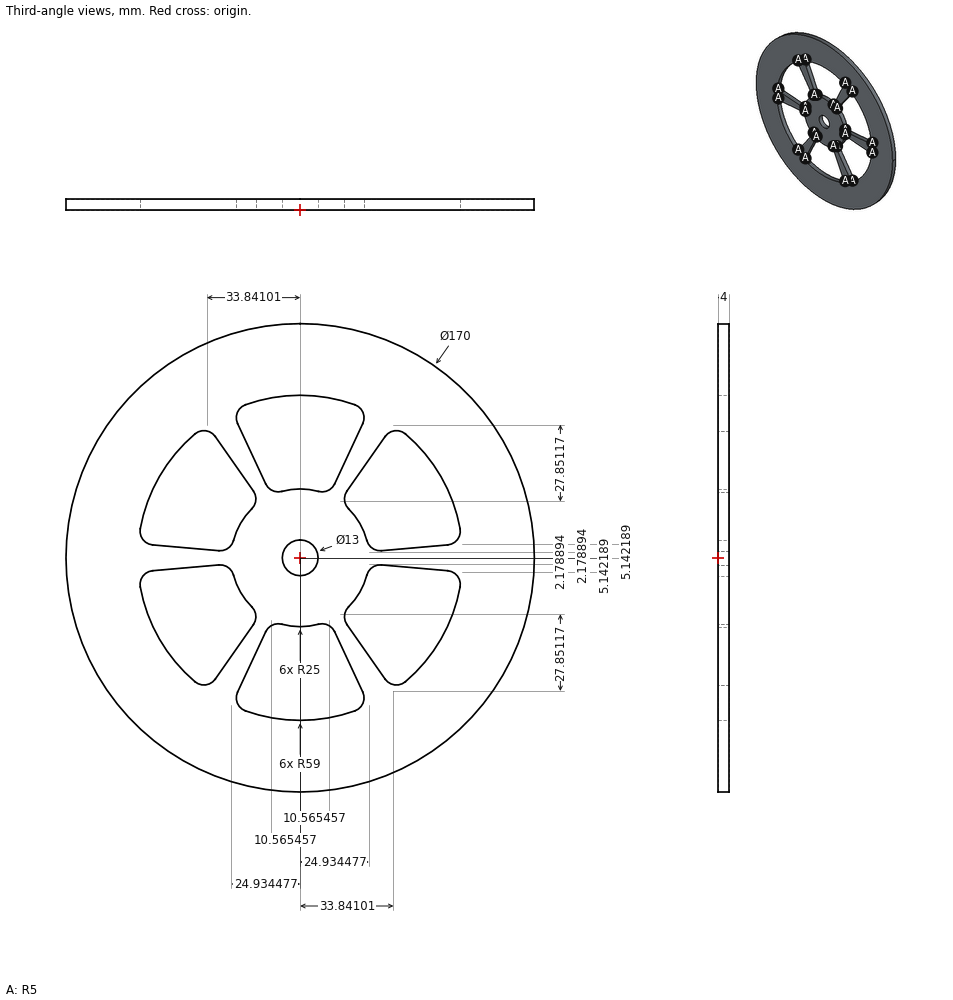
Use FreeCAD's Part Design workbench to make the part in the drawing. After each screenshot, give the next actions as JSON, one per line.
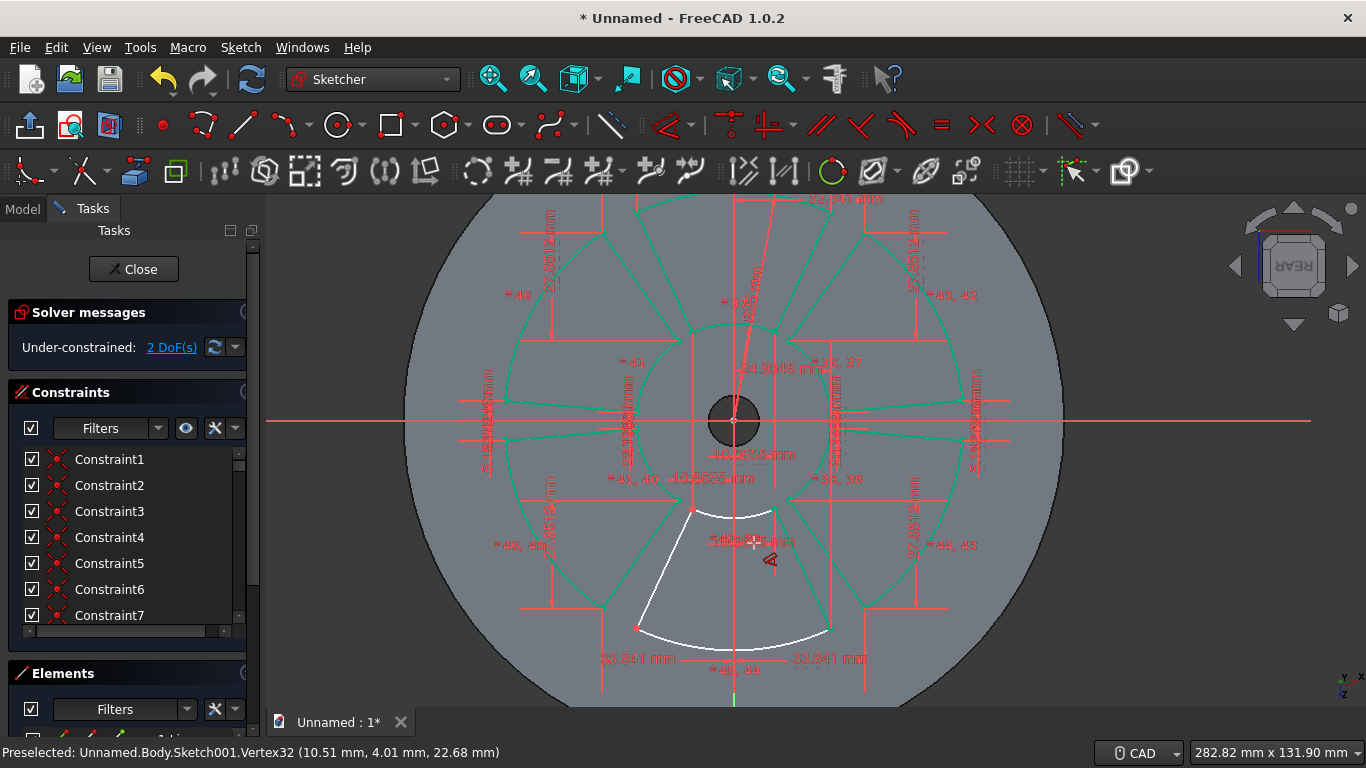
{"action": "left_click", "coordinate": [693, 509]}
{"action": "left_click", "coordinate": [704, 387]}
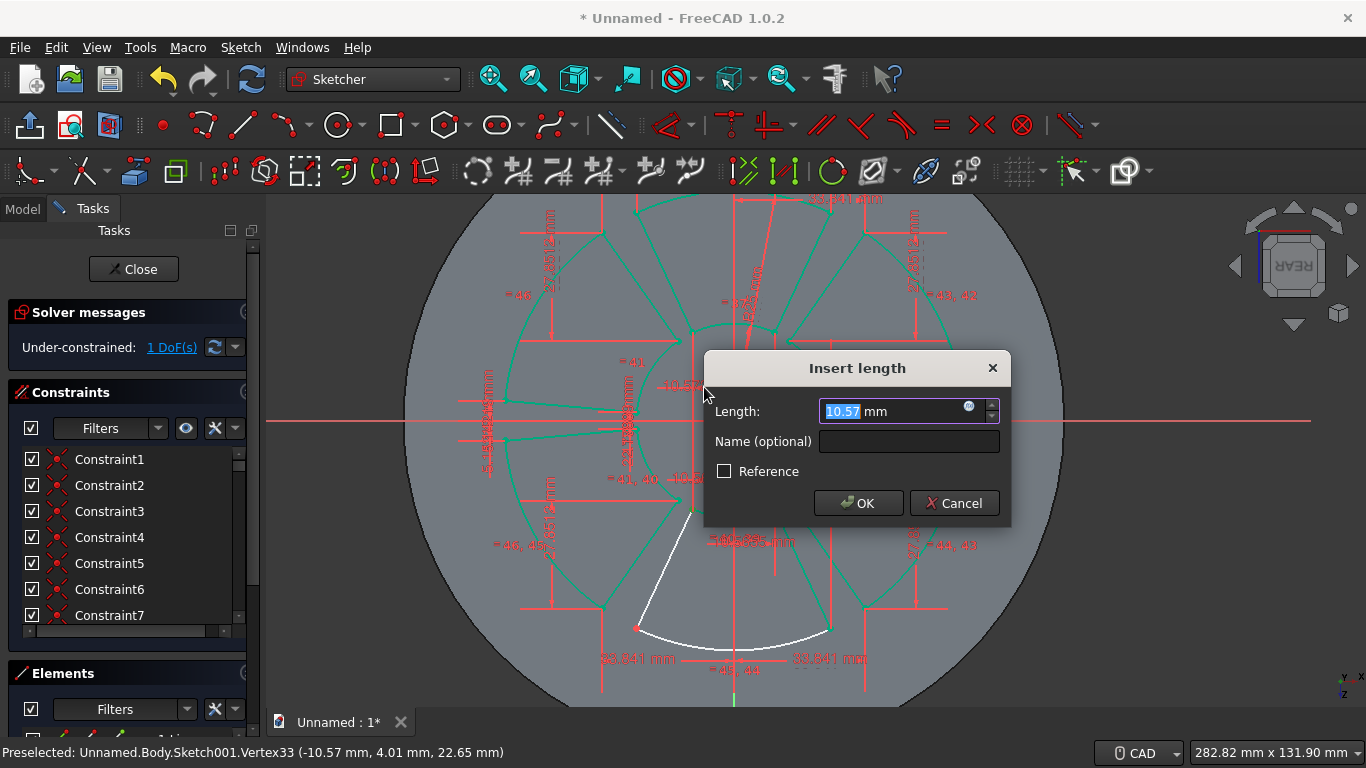
{"action": "type", "text": "10.565457"}
{"action": "key", "text": "Return"}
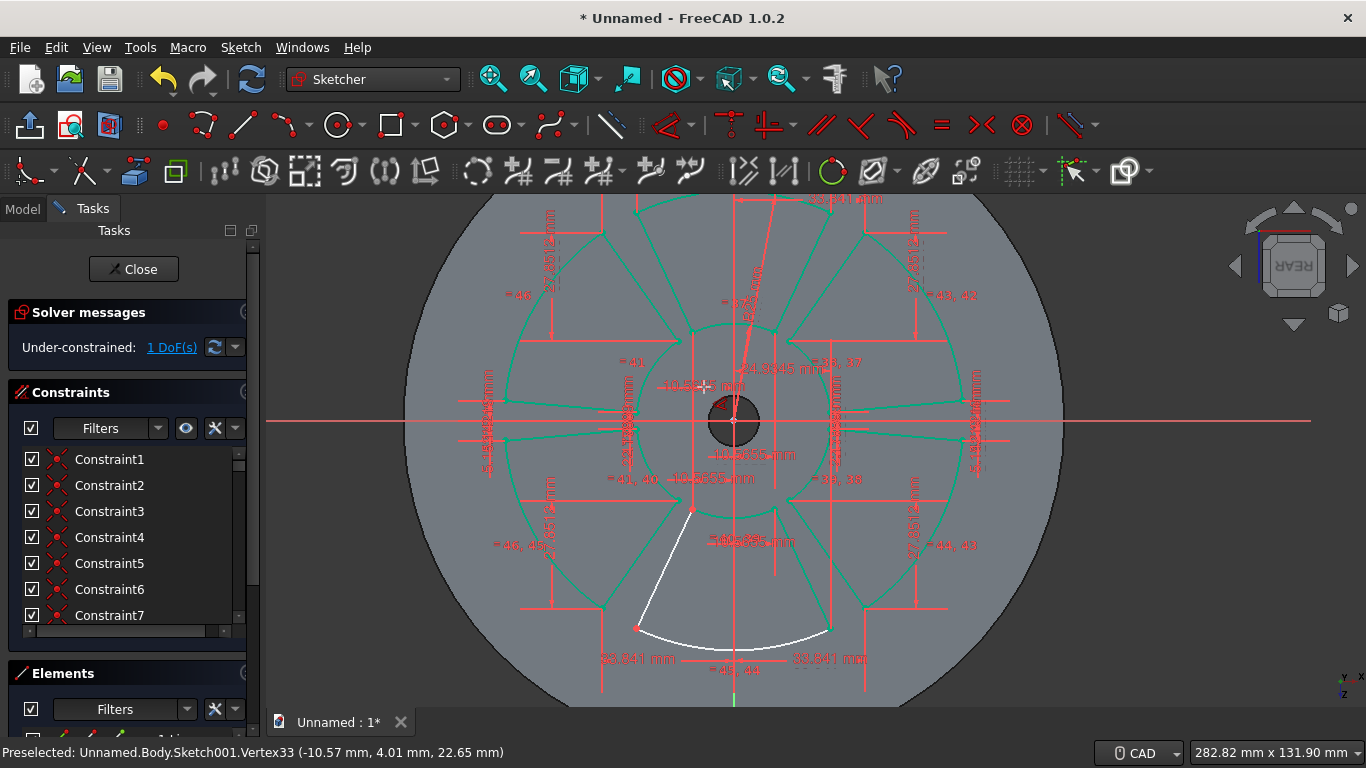
{"action": "left_click", "coordinate": [637, 629]}
{"action": "left_click", "coordinate": [708, 663]}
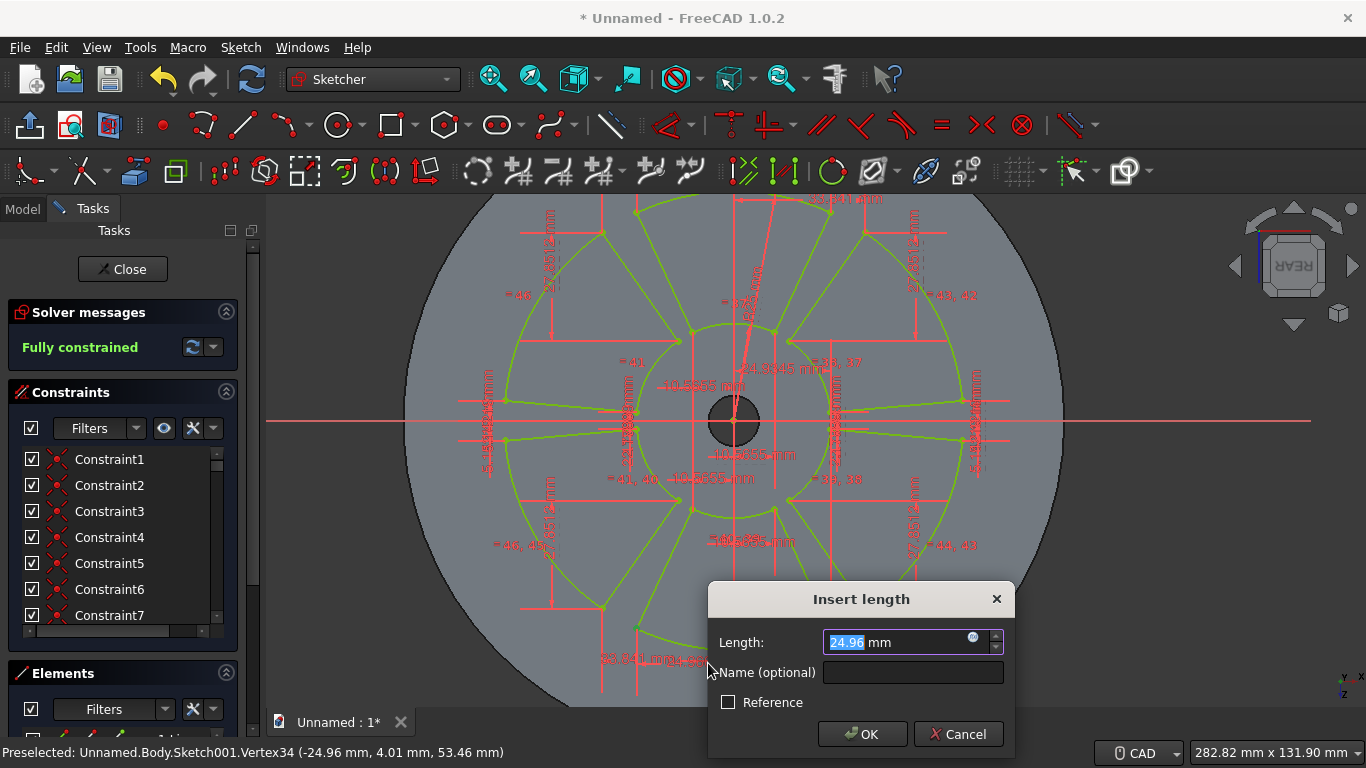
{"action": "type", "text": "24.934477"}
{"action": "key", "text": "Return"}
{"action": "key", "text": "Escape"}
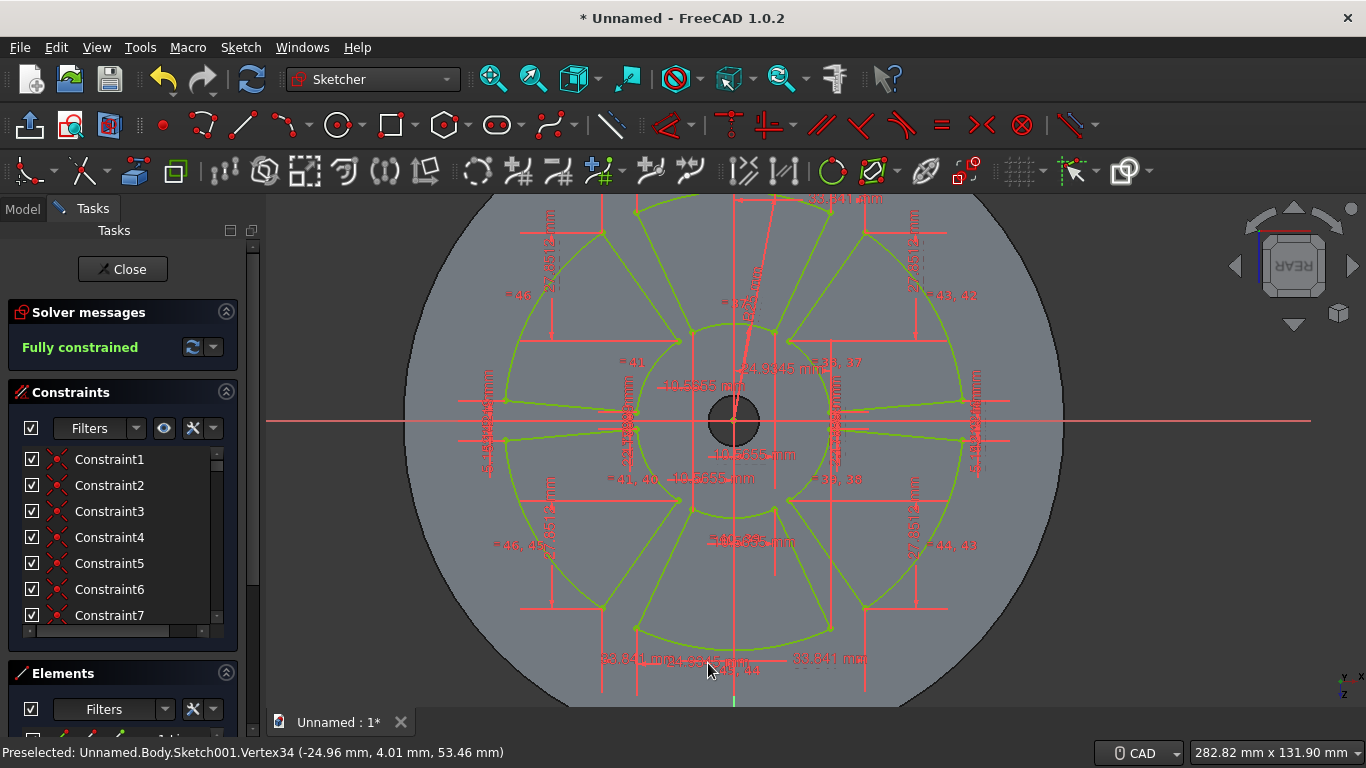
{"action": "left_click", "coordinate": [123, 269]}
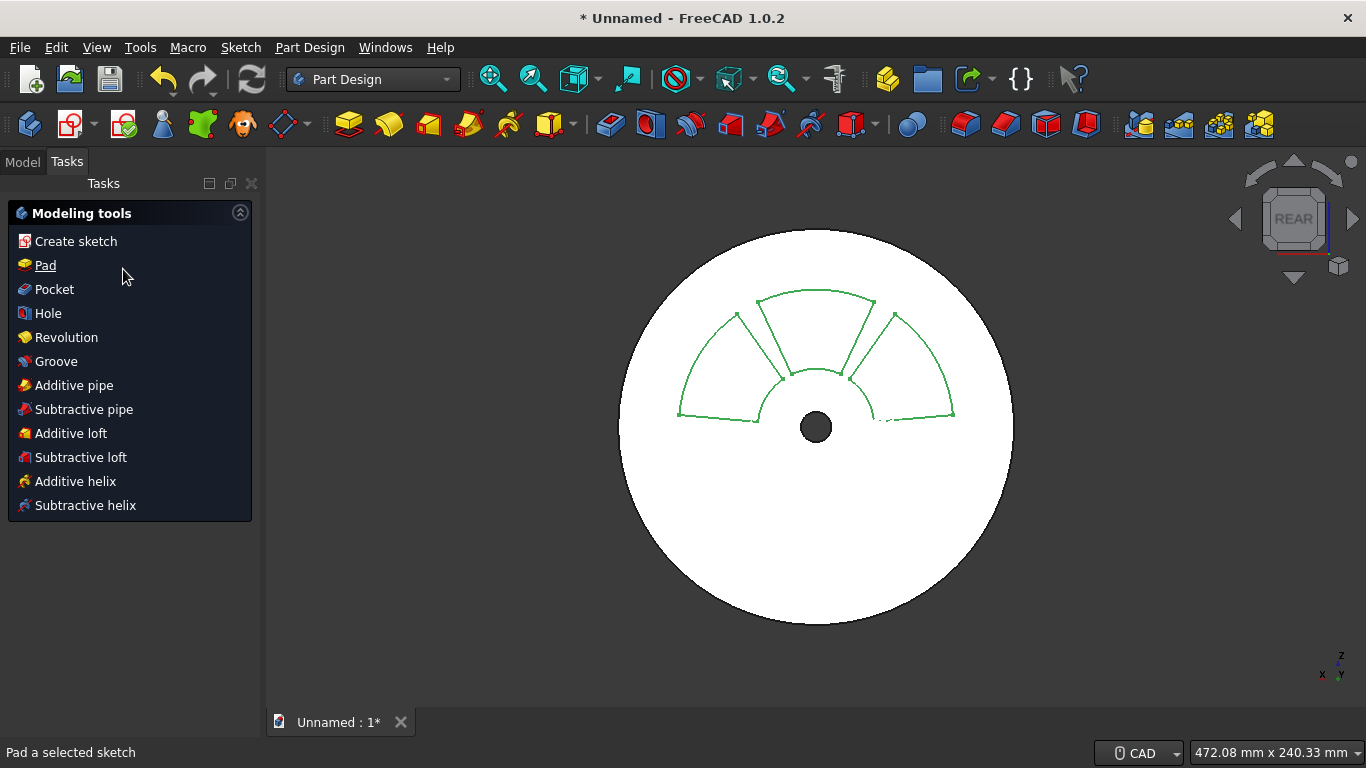
{"action": "left_click", "coordinate": [612, 124]}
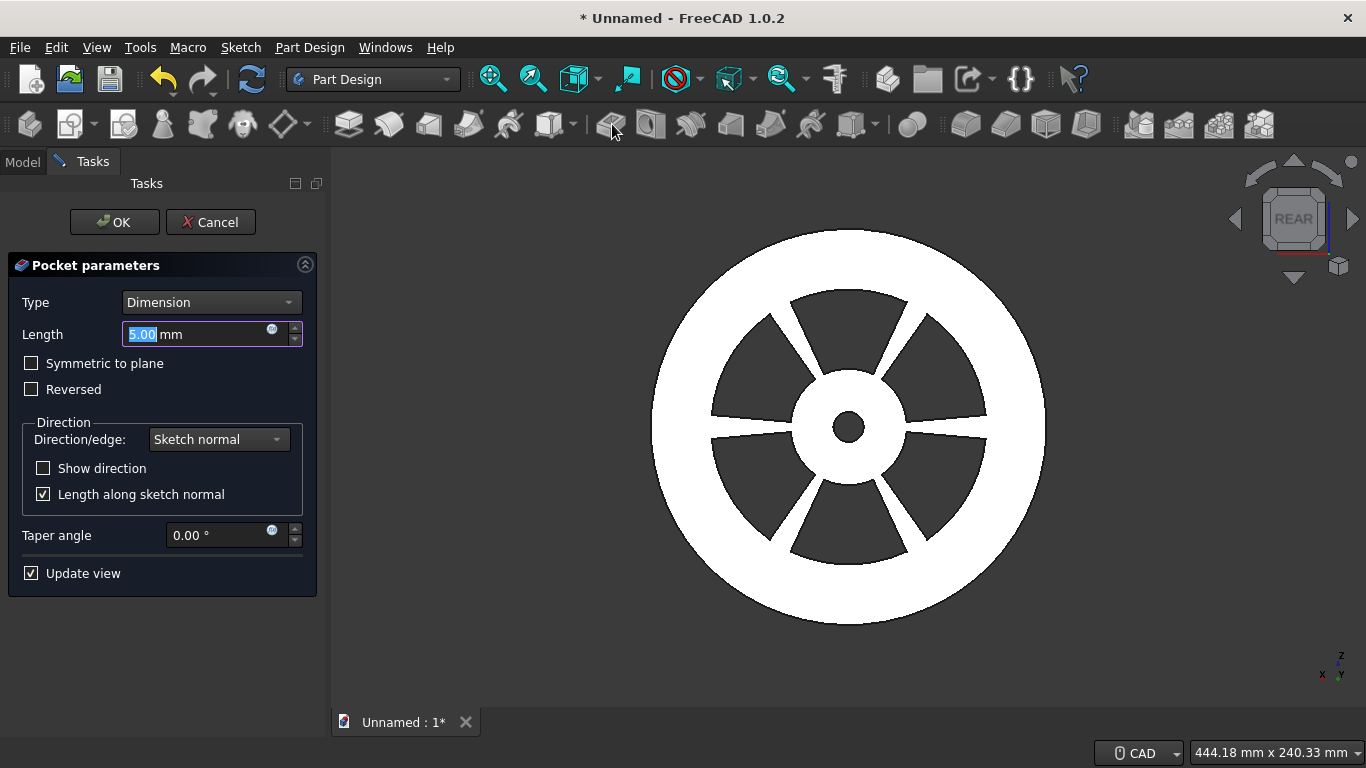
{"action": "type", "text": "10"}
{"action": "key", "text": "Tab"}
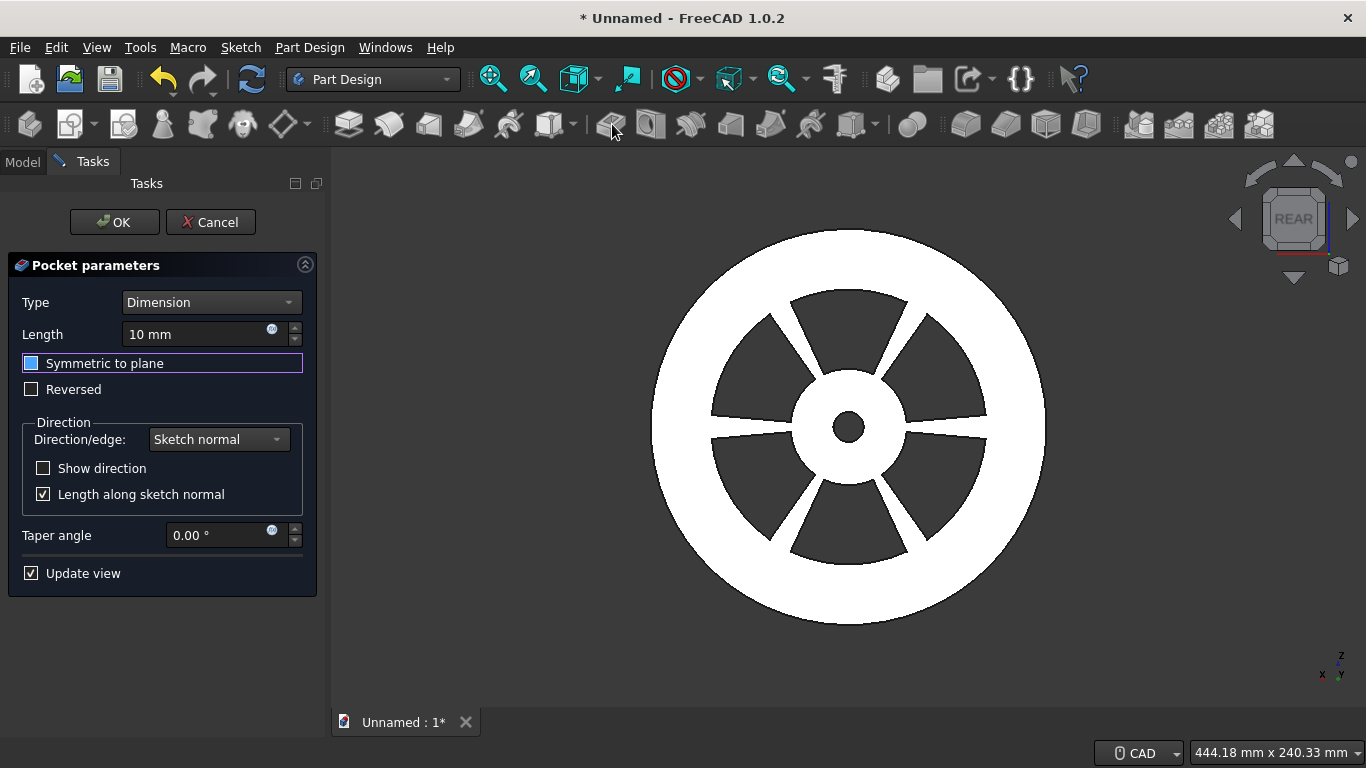
{"action": "left_click", "coordinate": [115, 222]}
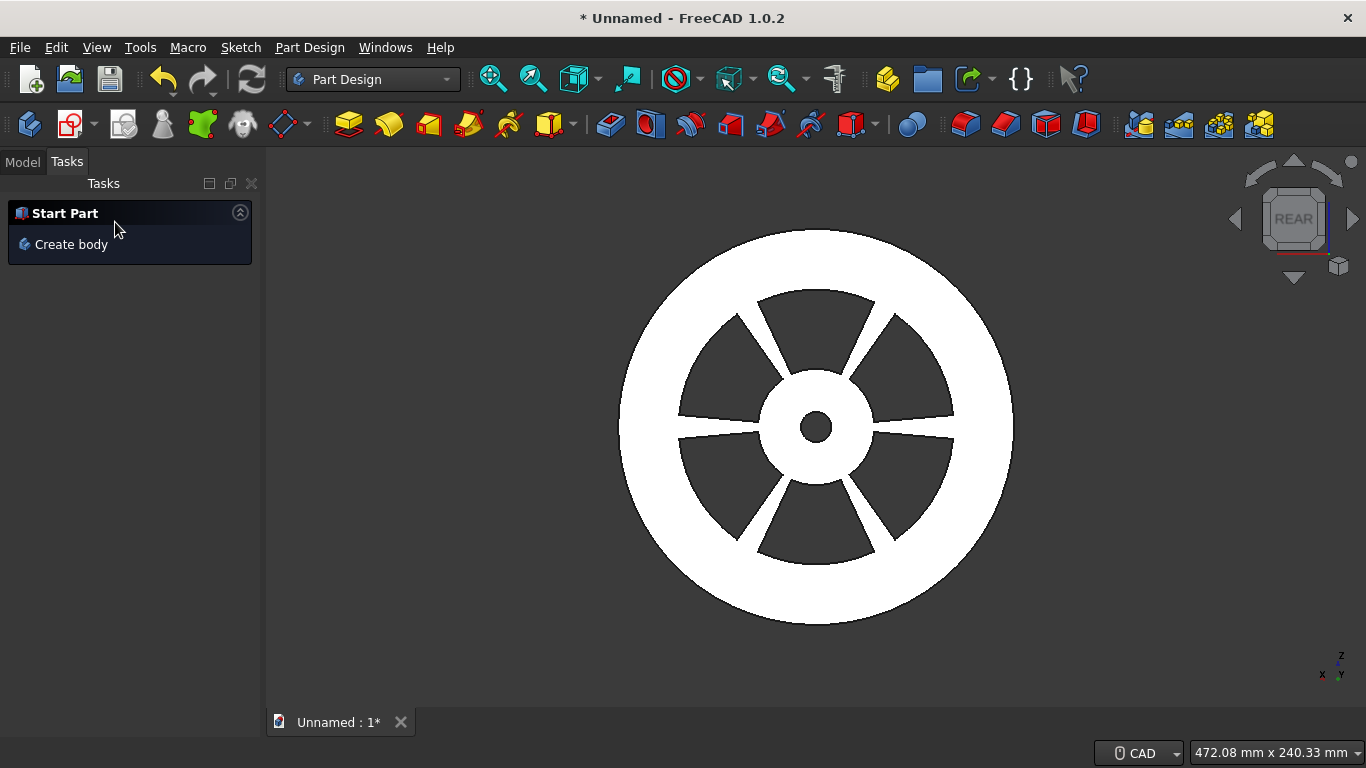
{"action": "scroll", "coordinate": [841, 373], "scroll_direction": "up", "scroll_amount": 8}